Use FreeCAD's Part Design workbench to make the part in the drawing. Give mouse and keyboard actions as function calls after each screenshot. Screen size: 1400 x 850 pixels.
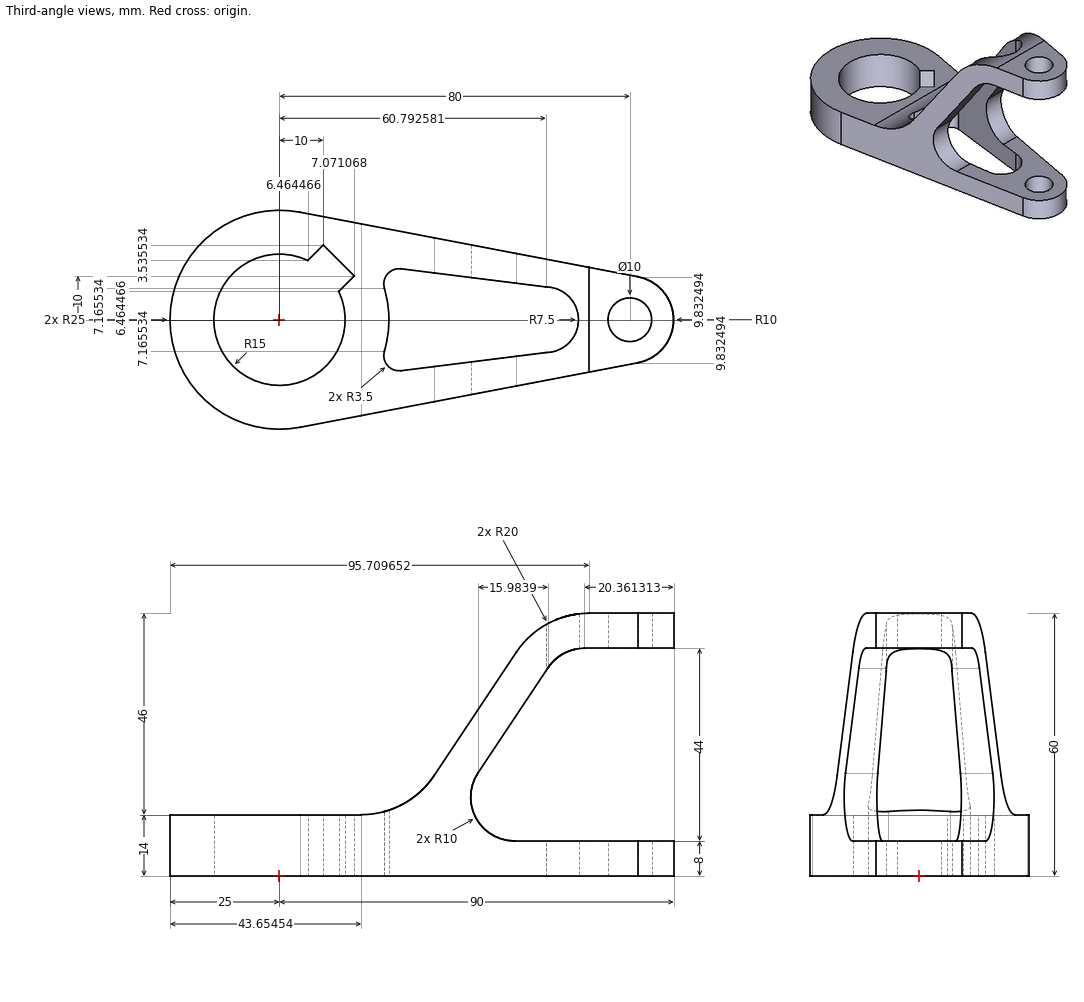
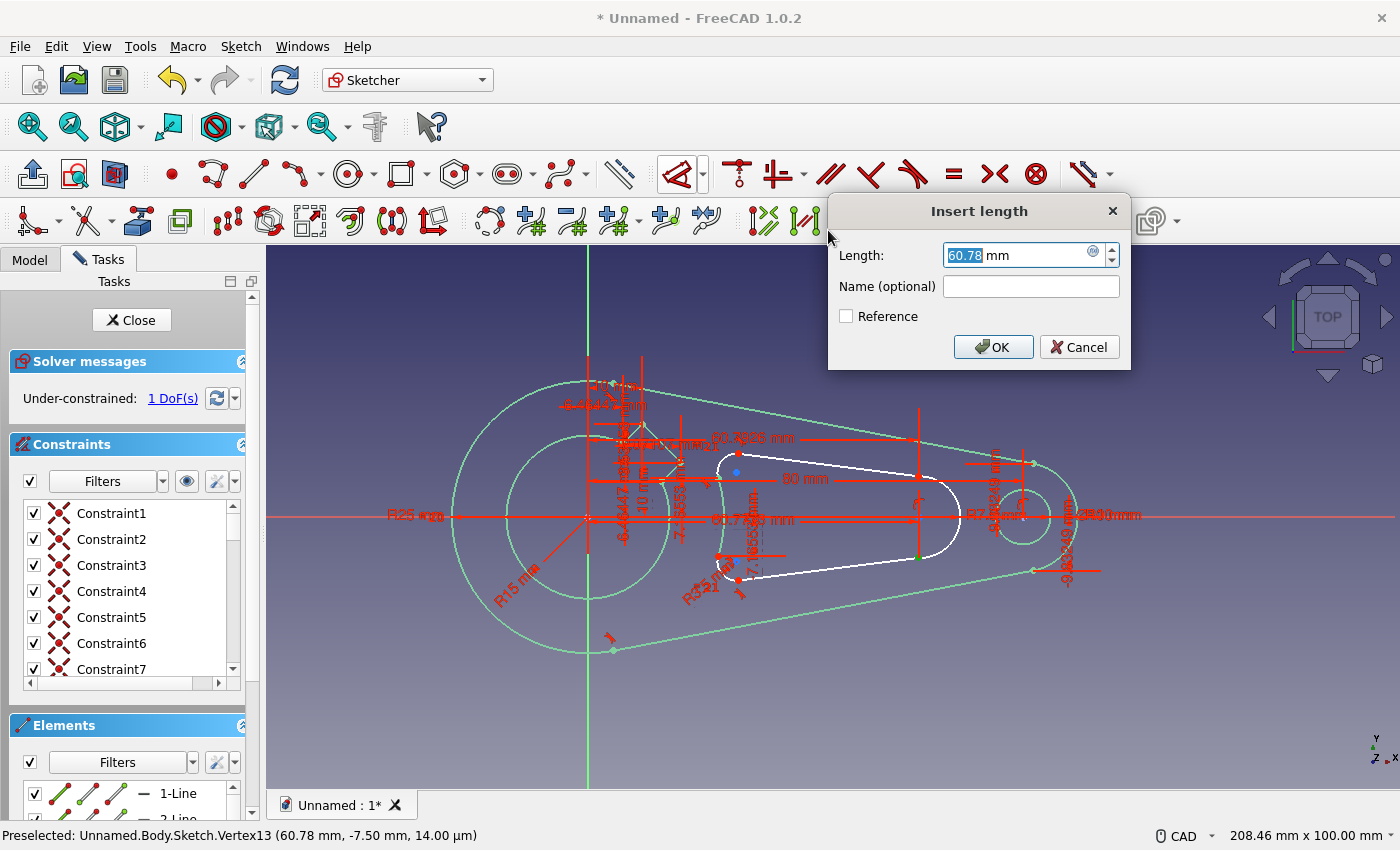
text(60.792581)
key(Return)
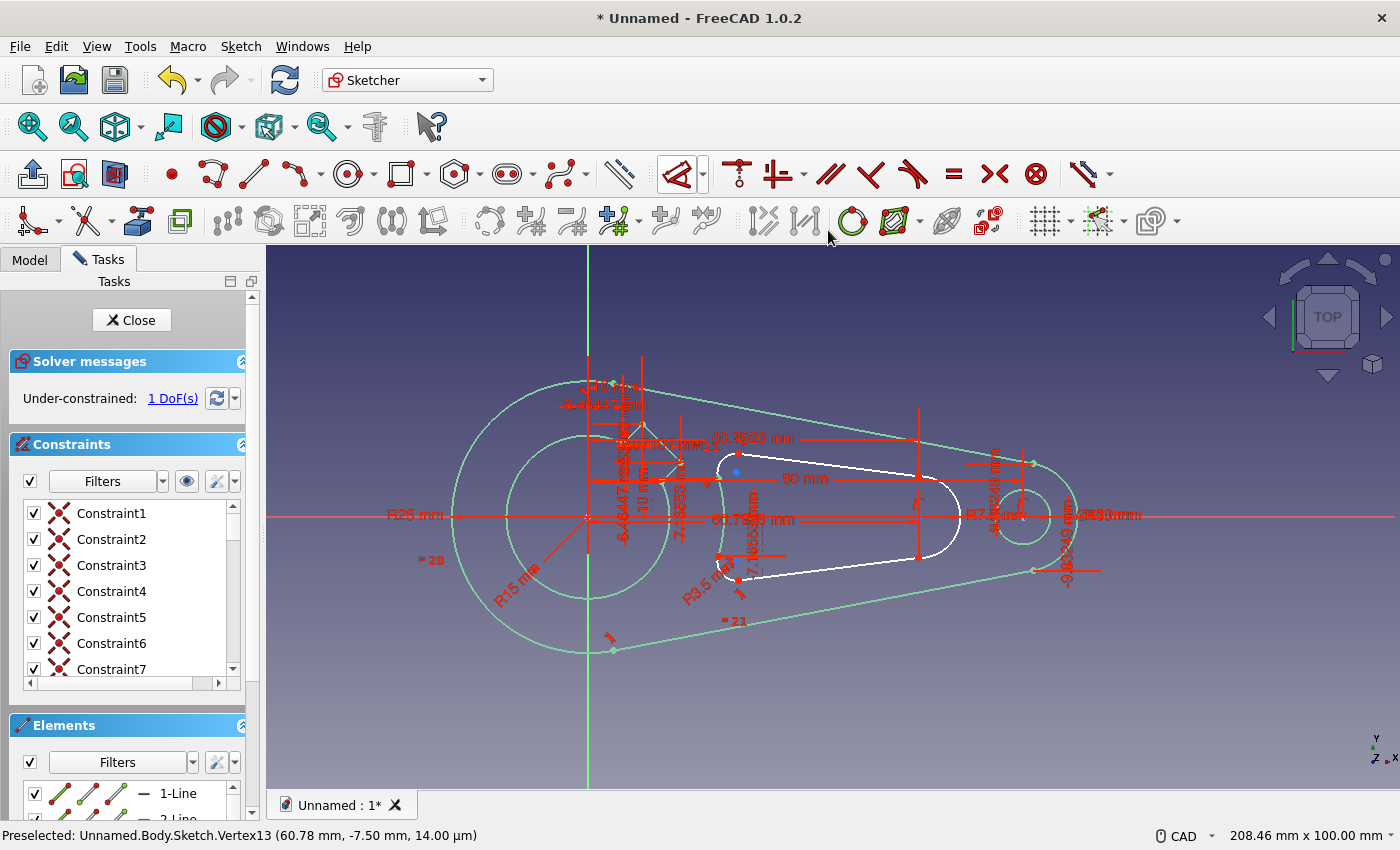
click(920, 517)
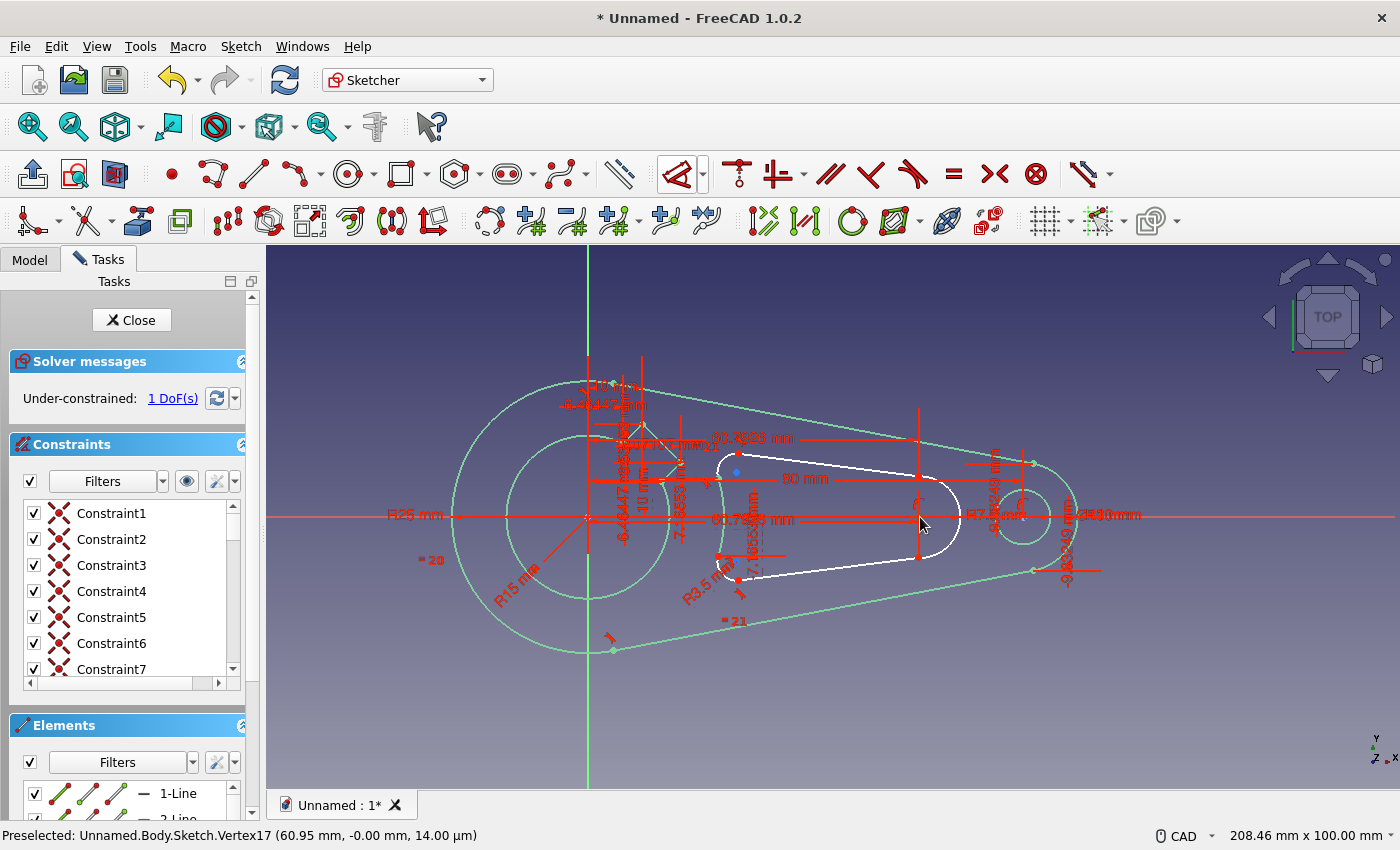
click(702, 174)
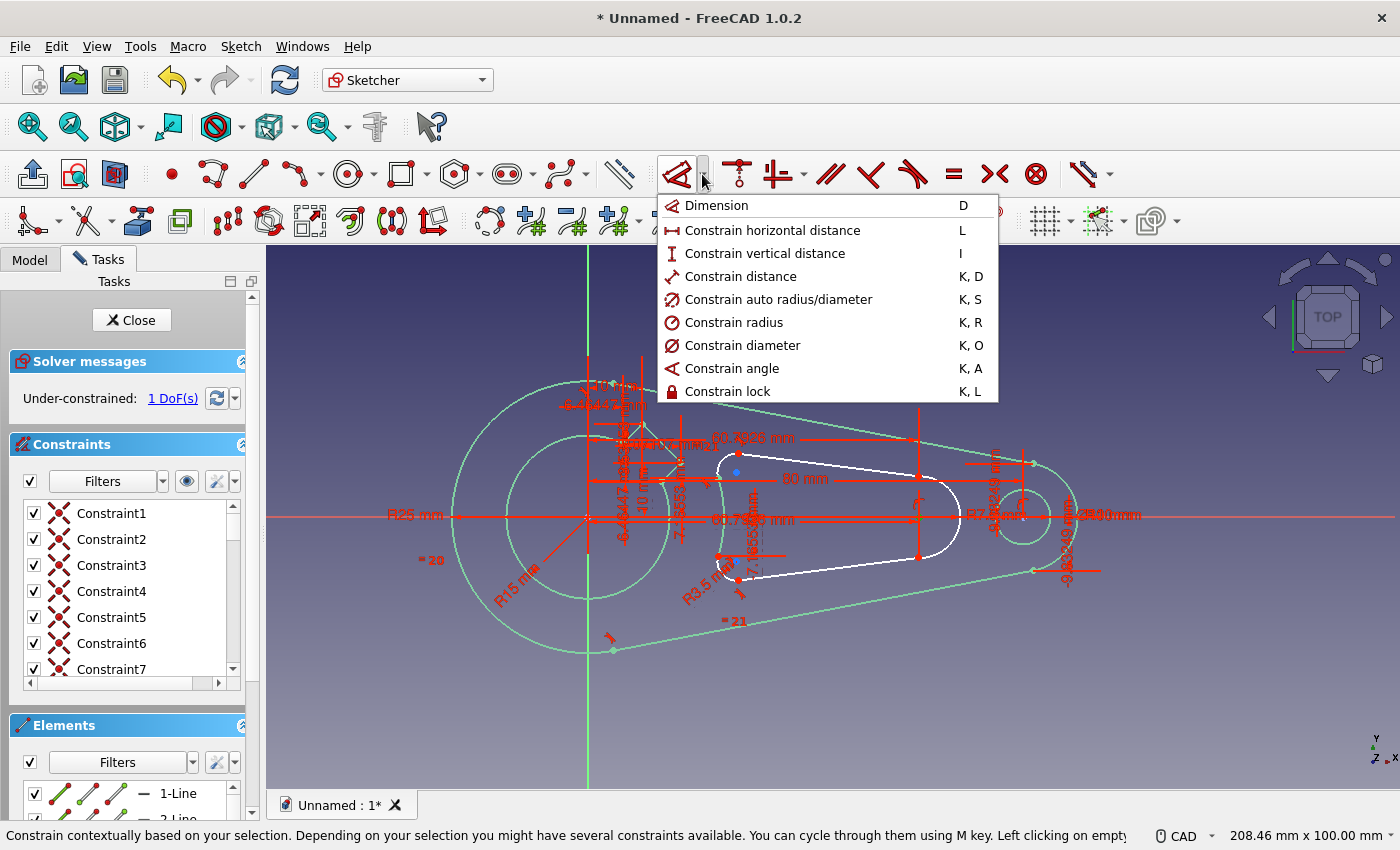
click(828, 230)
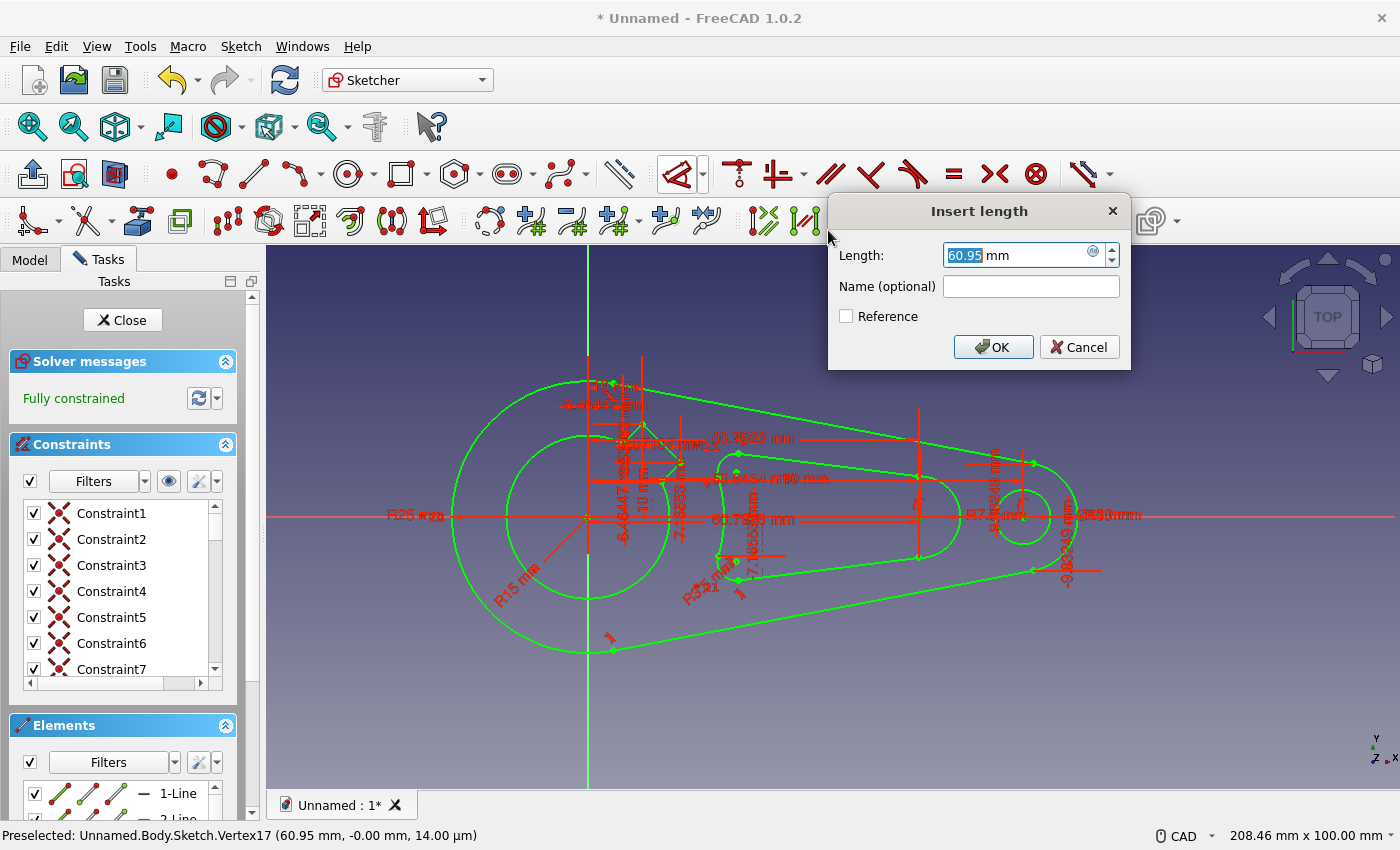
text(60.792581)
key(Return)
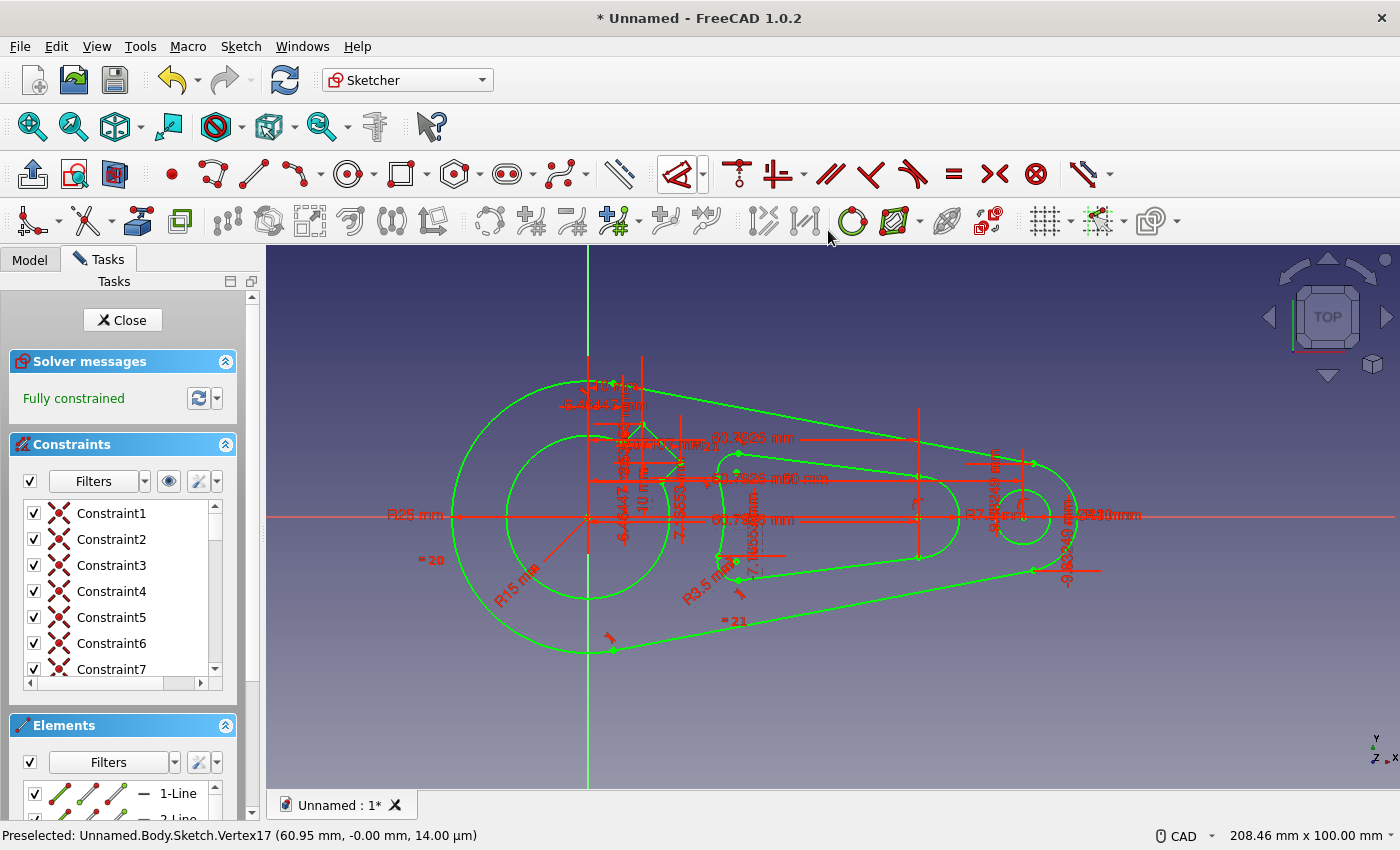
click(123, 320)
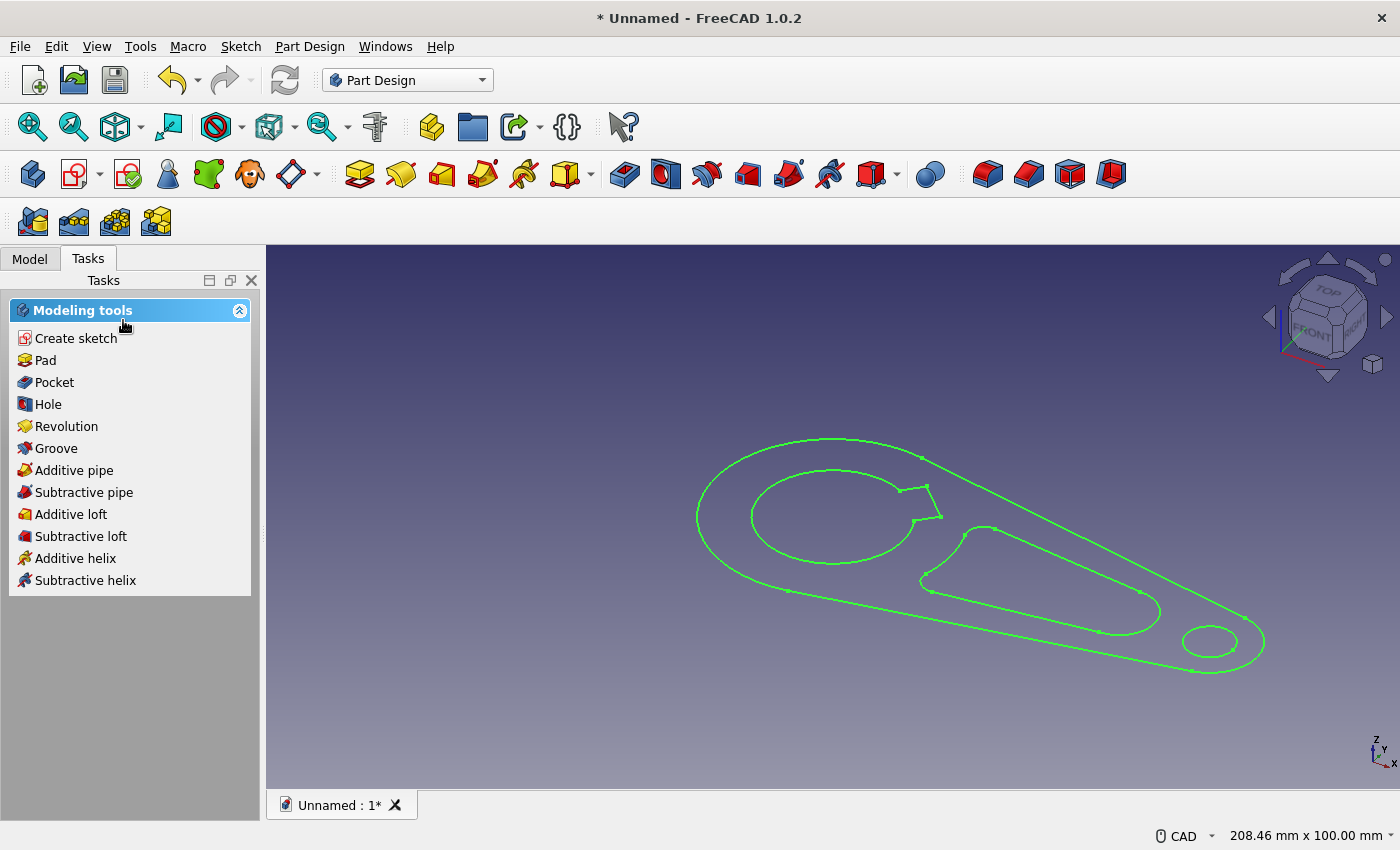
click(360, 174)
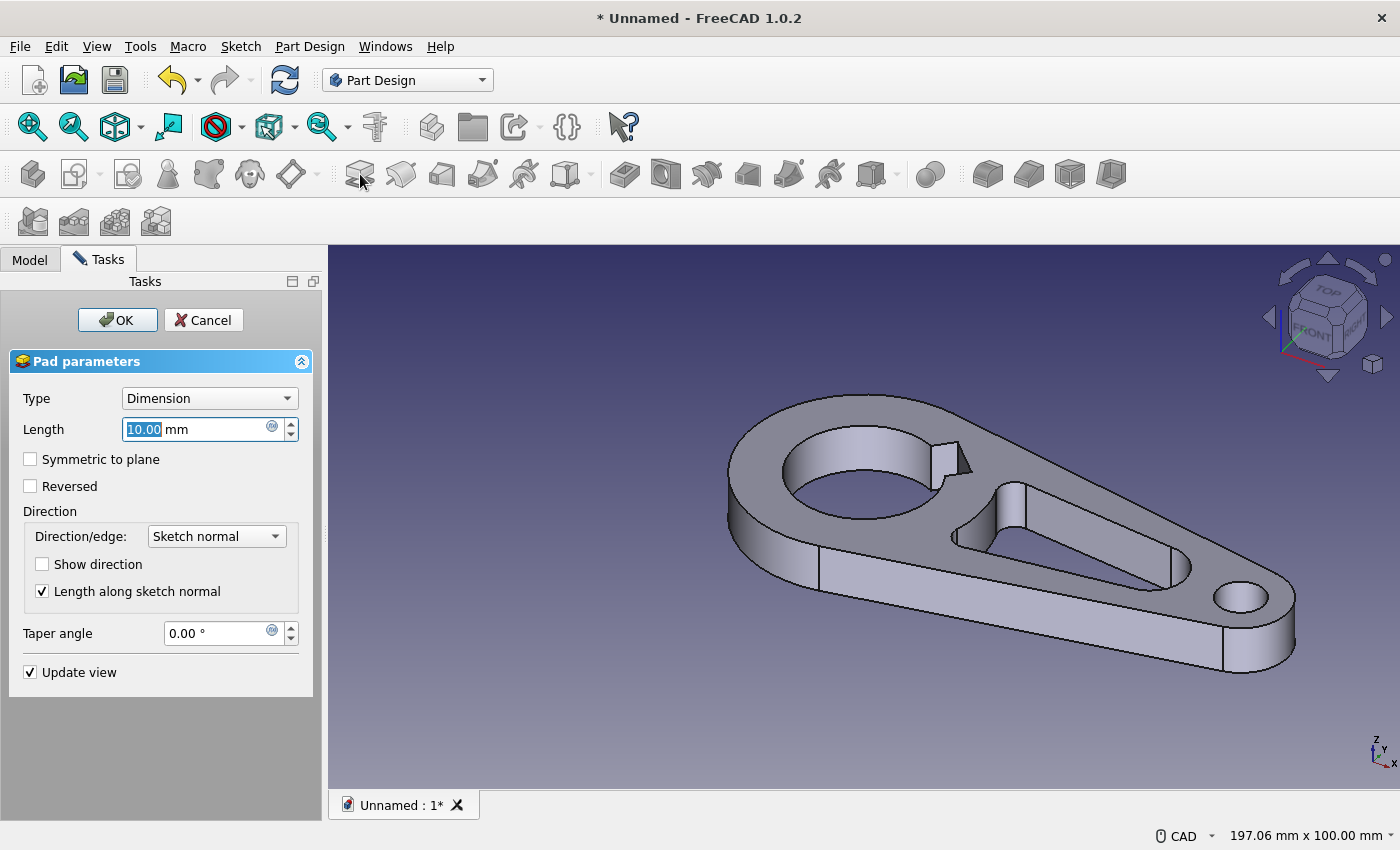
text(60)
key(Tab)